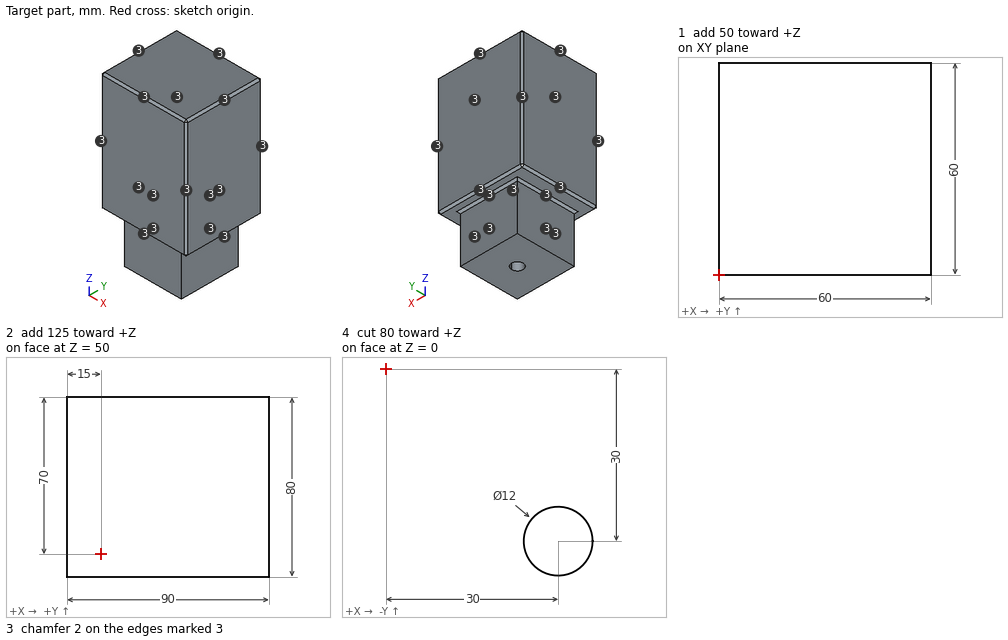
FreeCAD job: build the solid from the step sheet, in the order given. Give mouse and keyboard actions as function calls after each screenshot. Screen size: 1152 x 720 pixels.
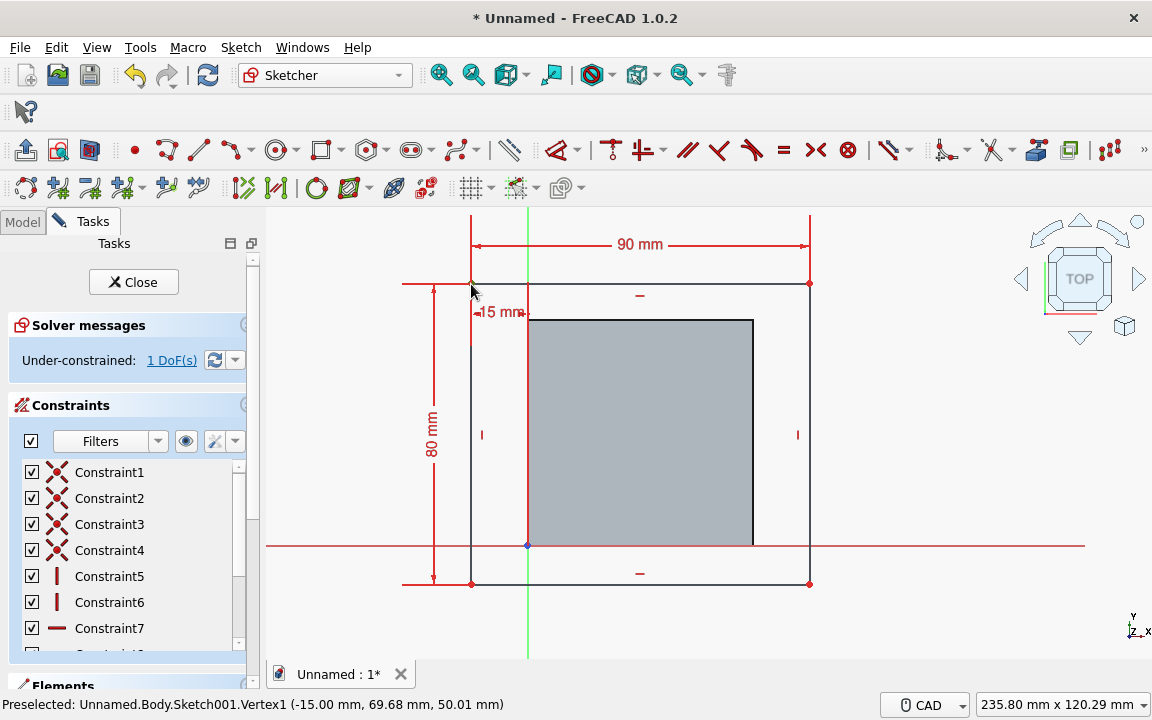
key(i)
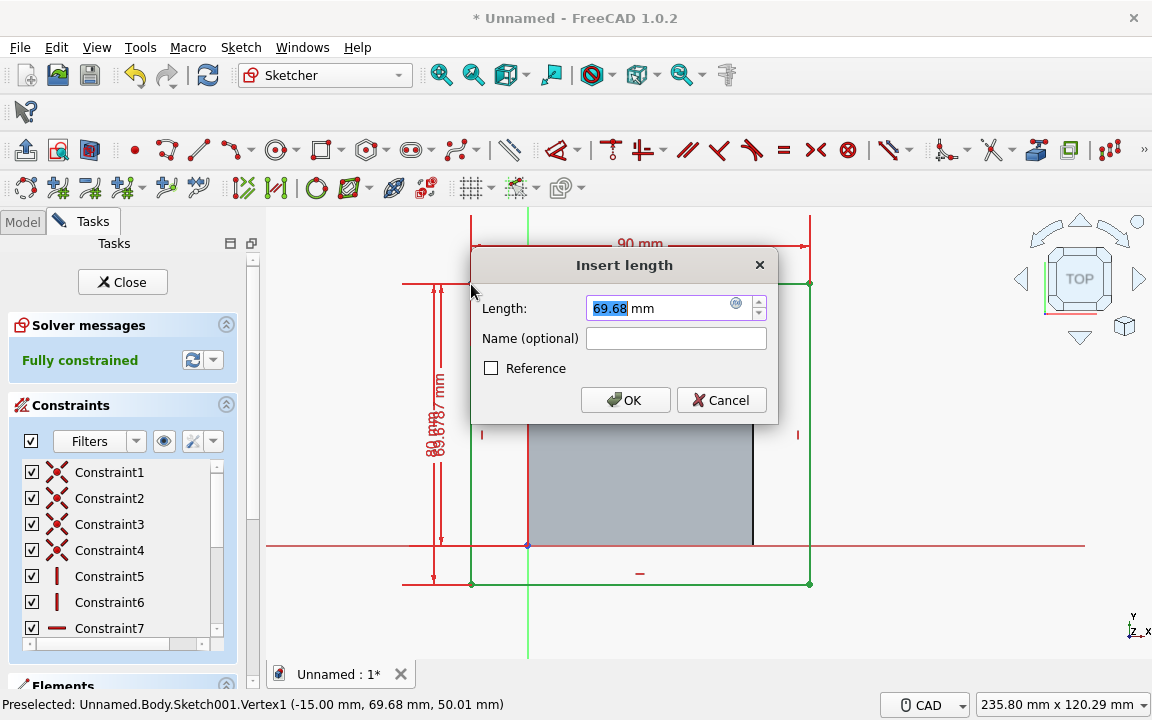
text(70)
key(Return)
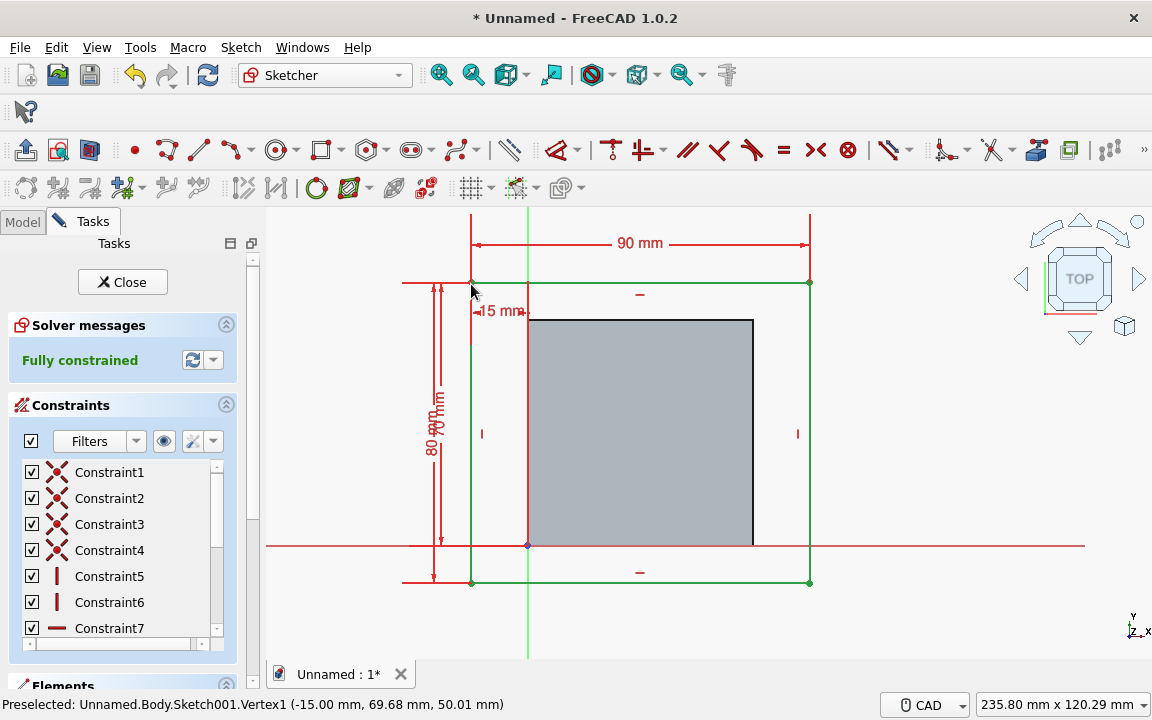
click(123, 282)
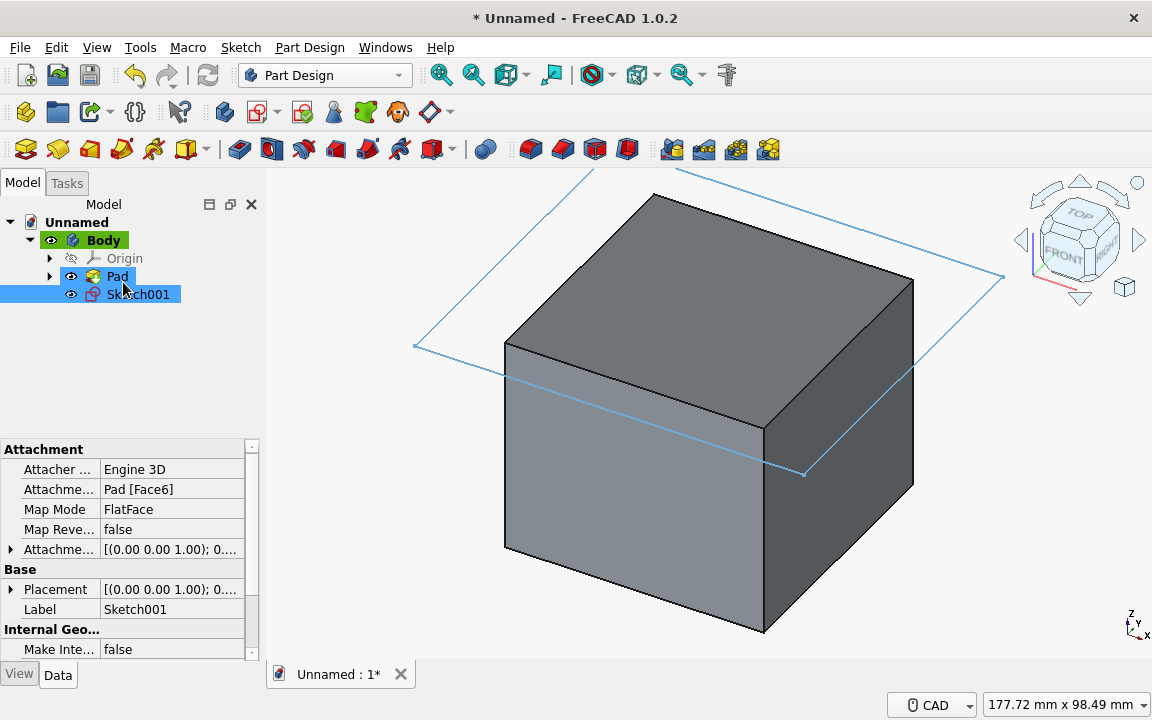
click(26, 150)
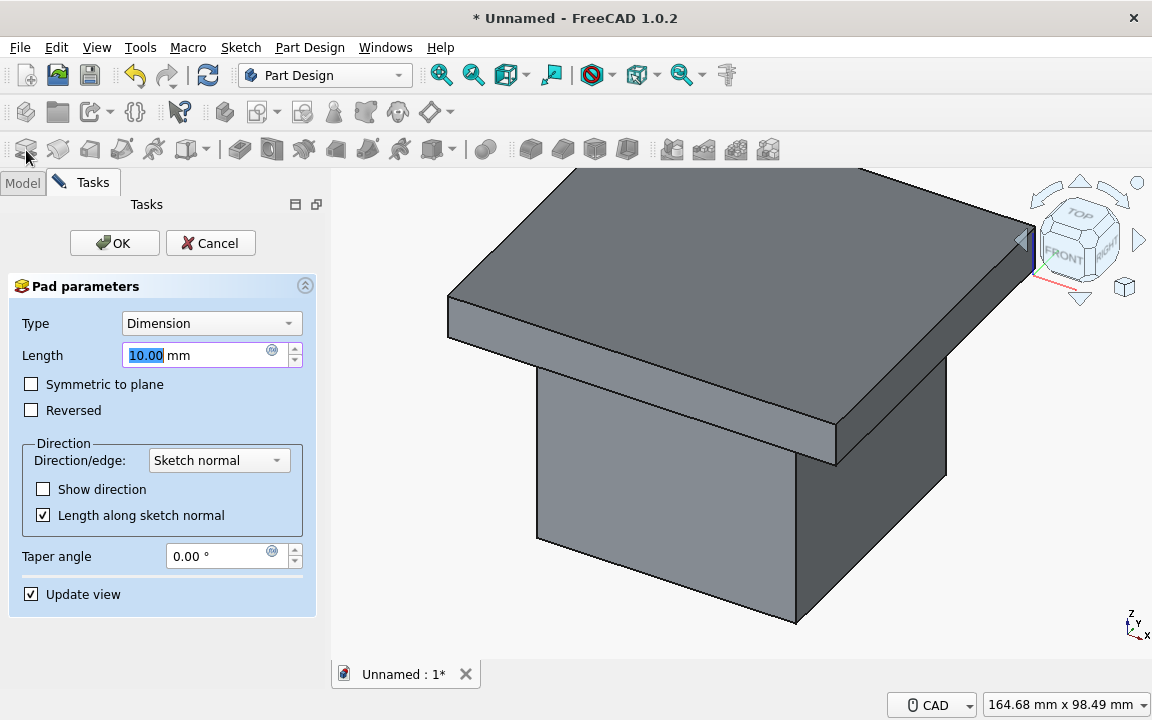
text(125)
key(Tab)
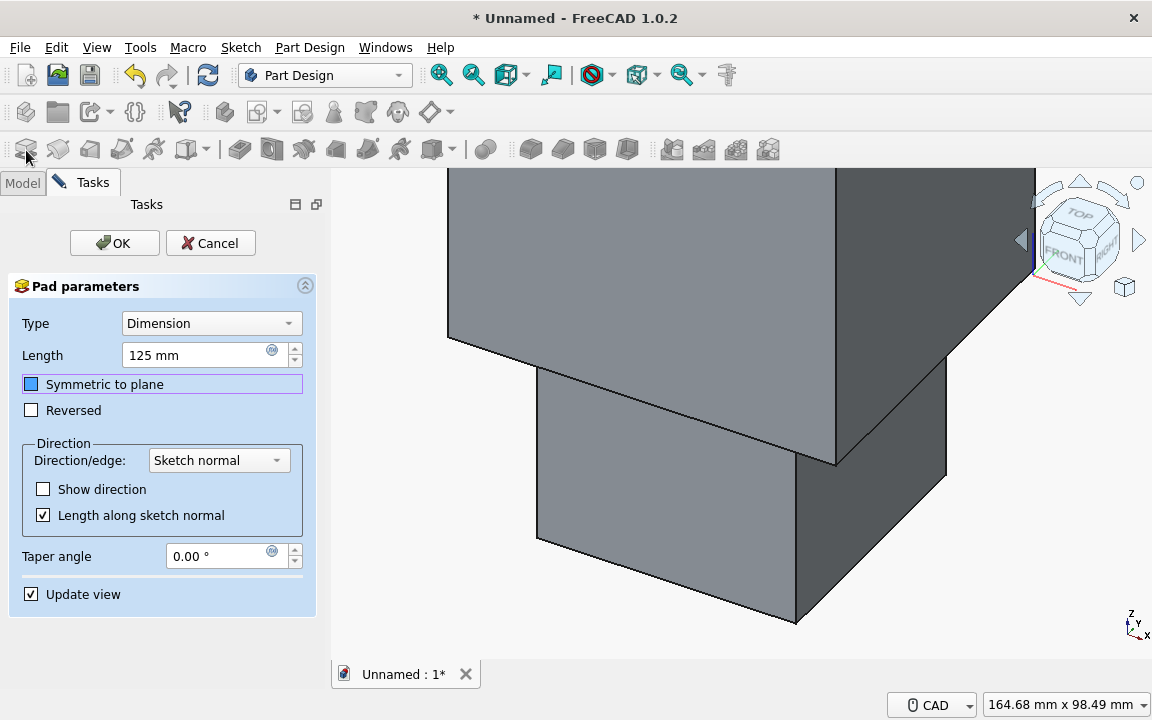
click(115, 243)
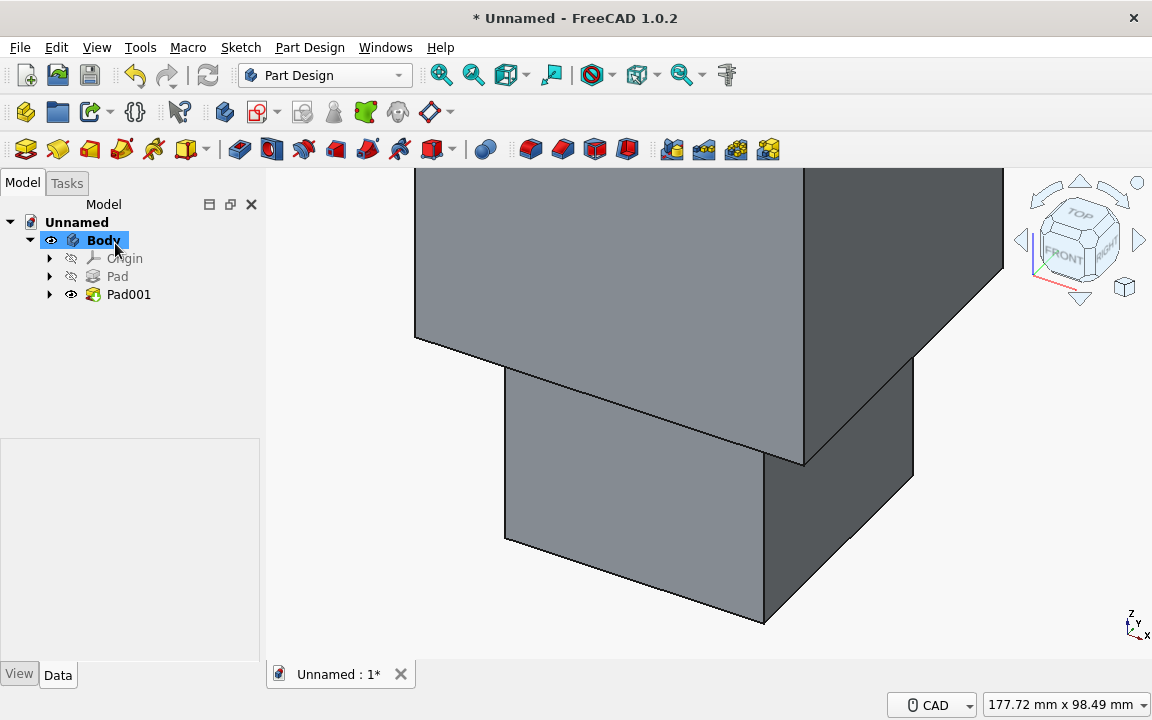
key(v)
key(f)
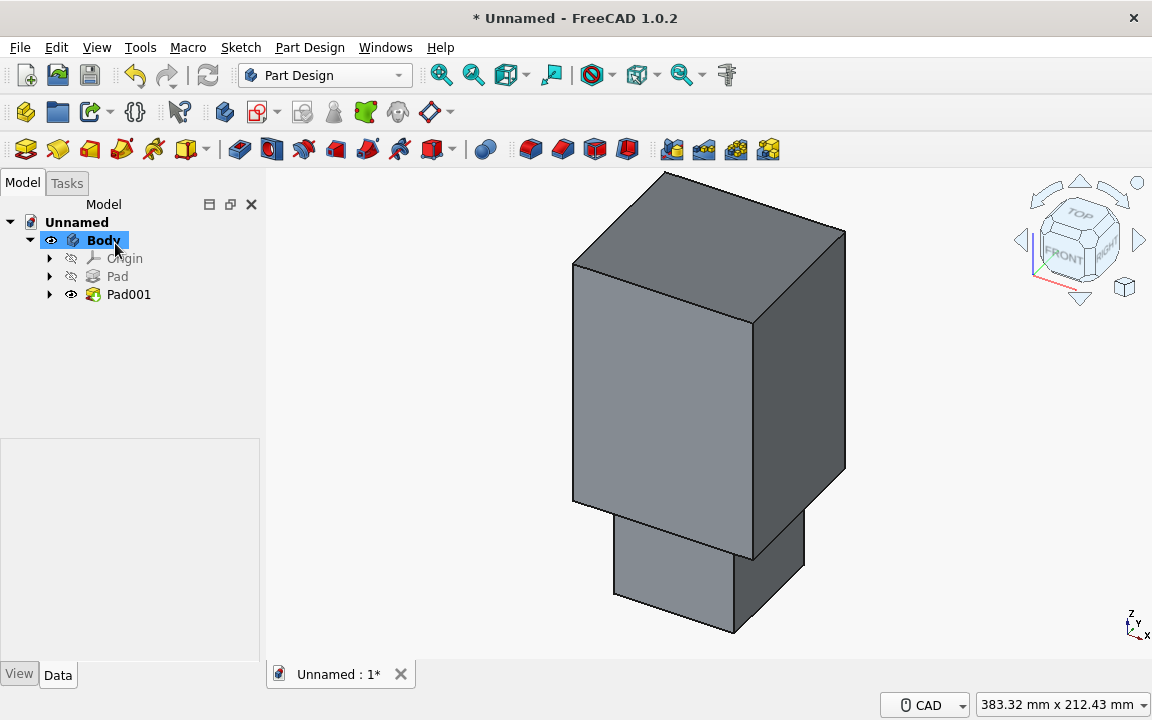
click(663, 411)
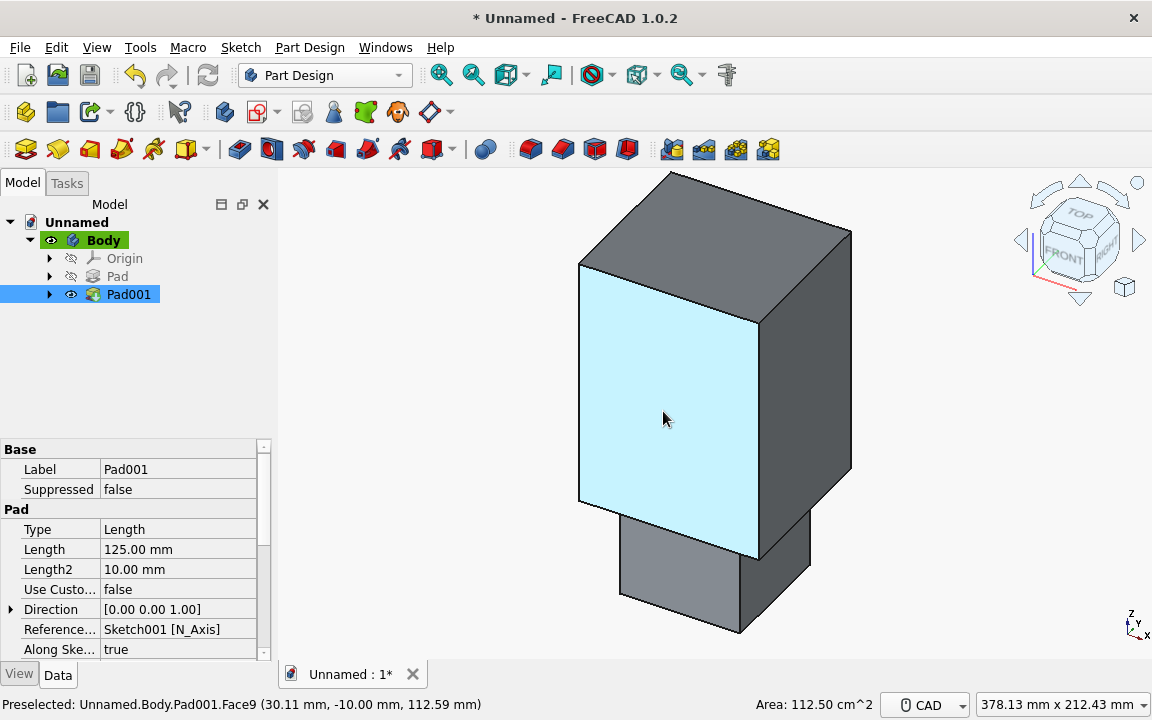
click(805, 277, ctrl)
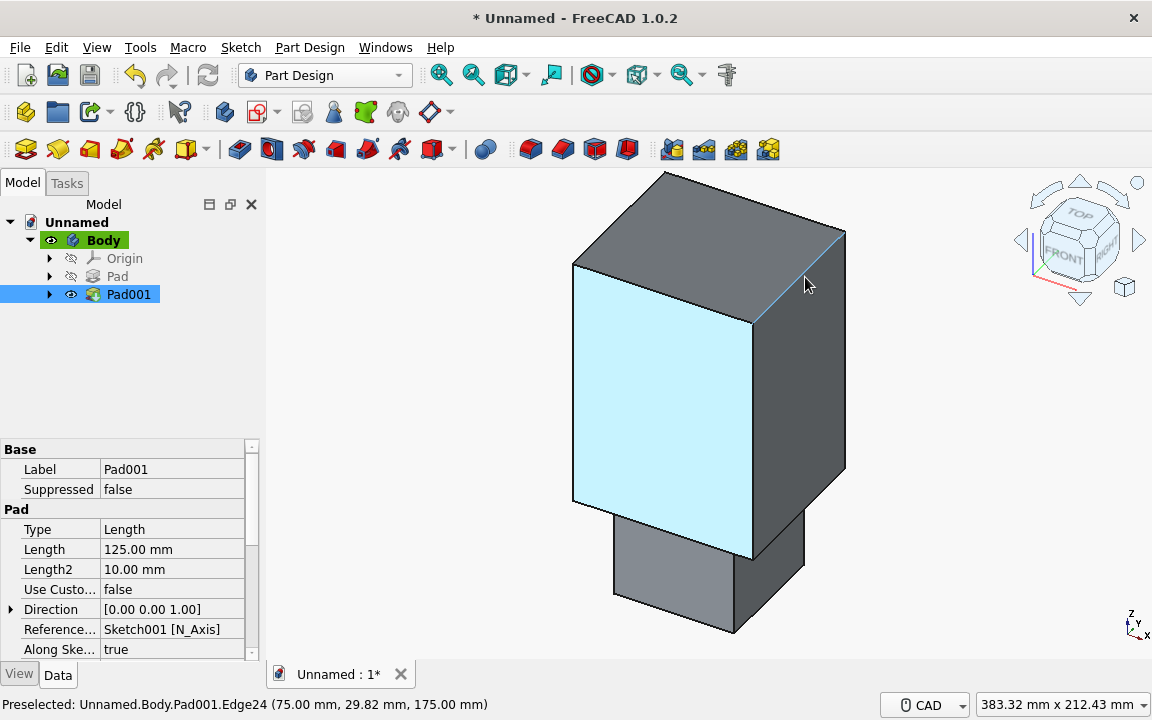
key(0)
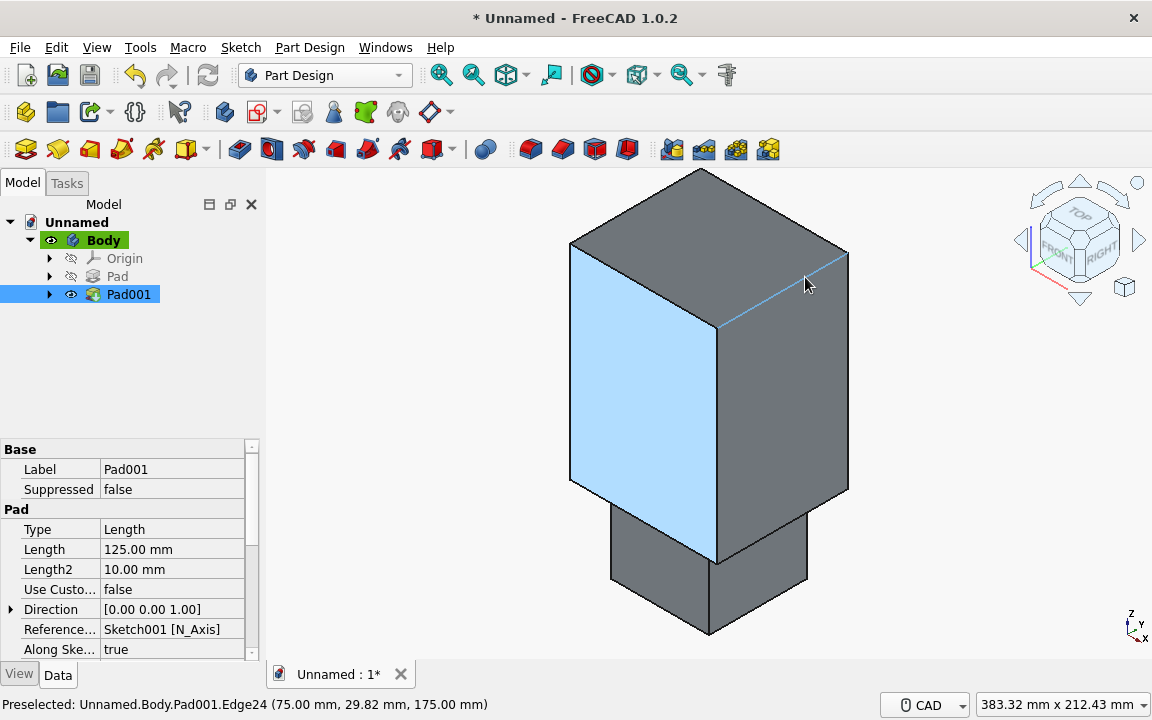
click(442, 76)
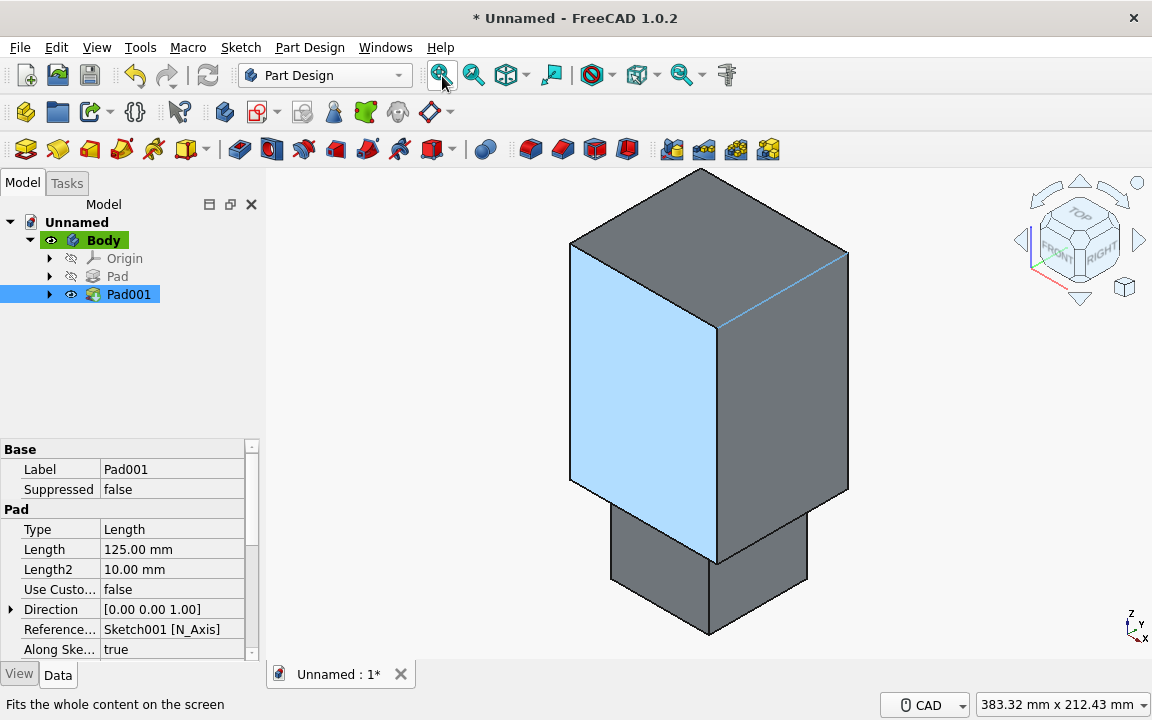
key(2)